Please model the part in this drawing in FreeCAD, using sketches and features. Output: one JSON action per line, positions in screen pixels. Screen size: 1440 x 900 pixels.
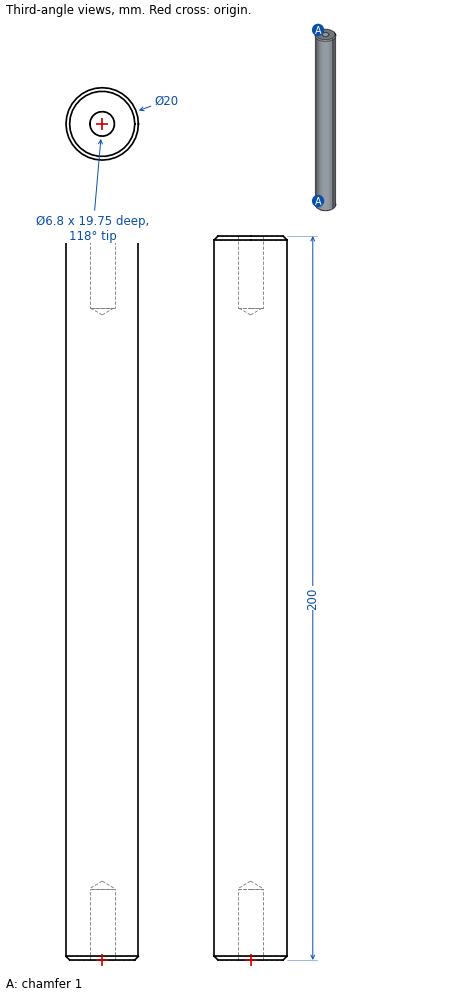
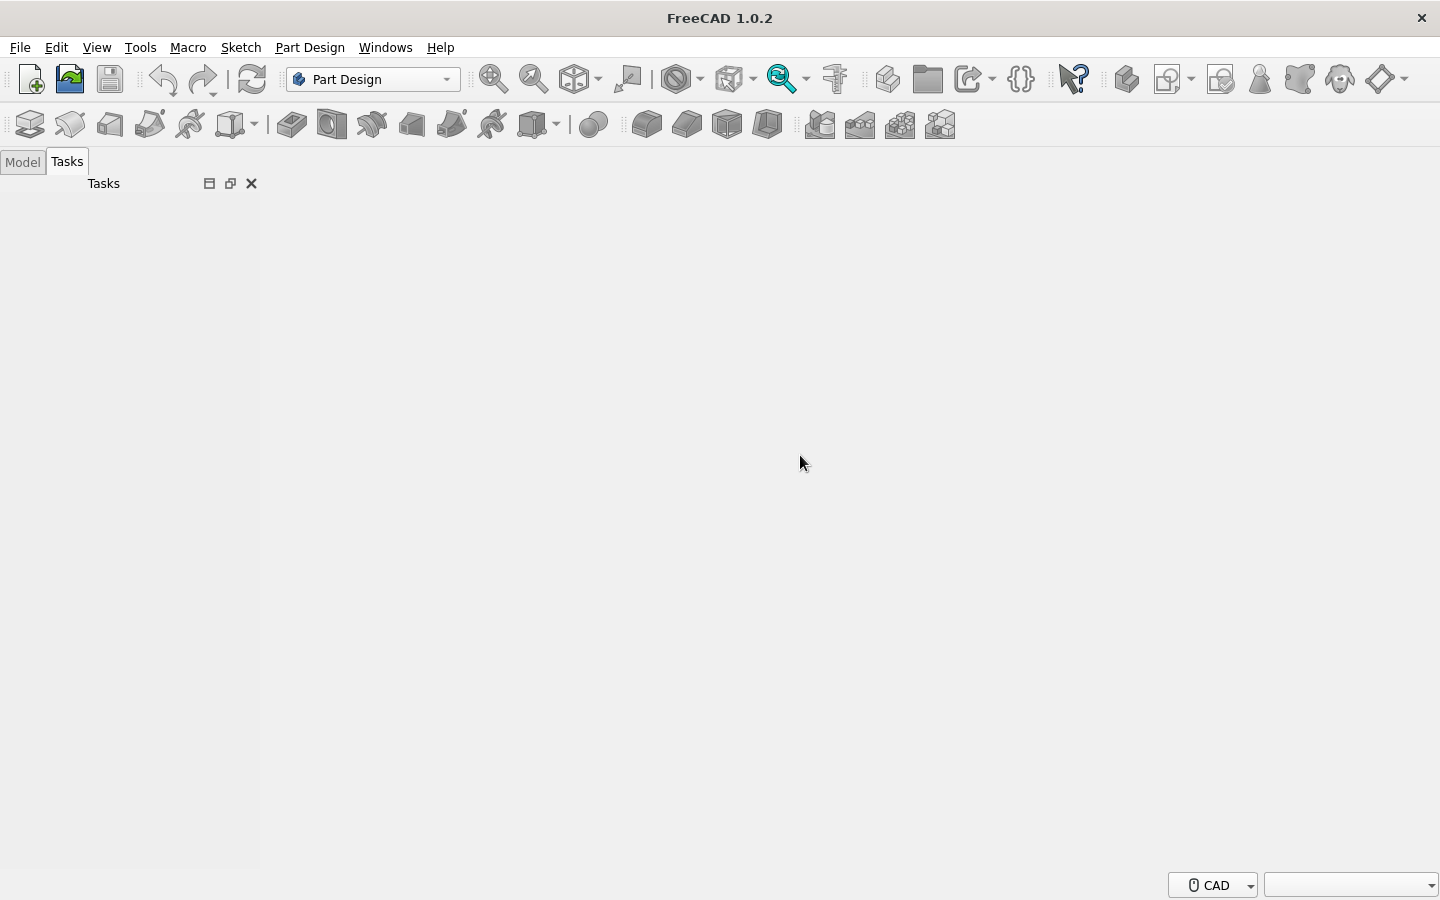
{"action": "key", "text": "ctrl+n"}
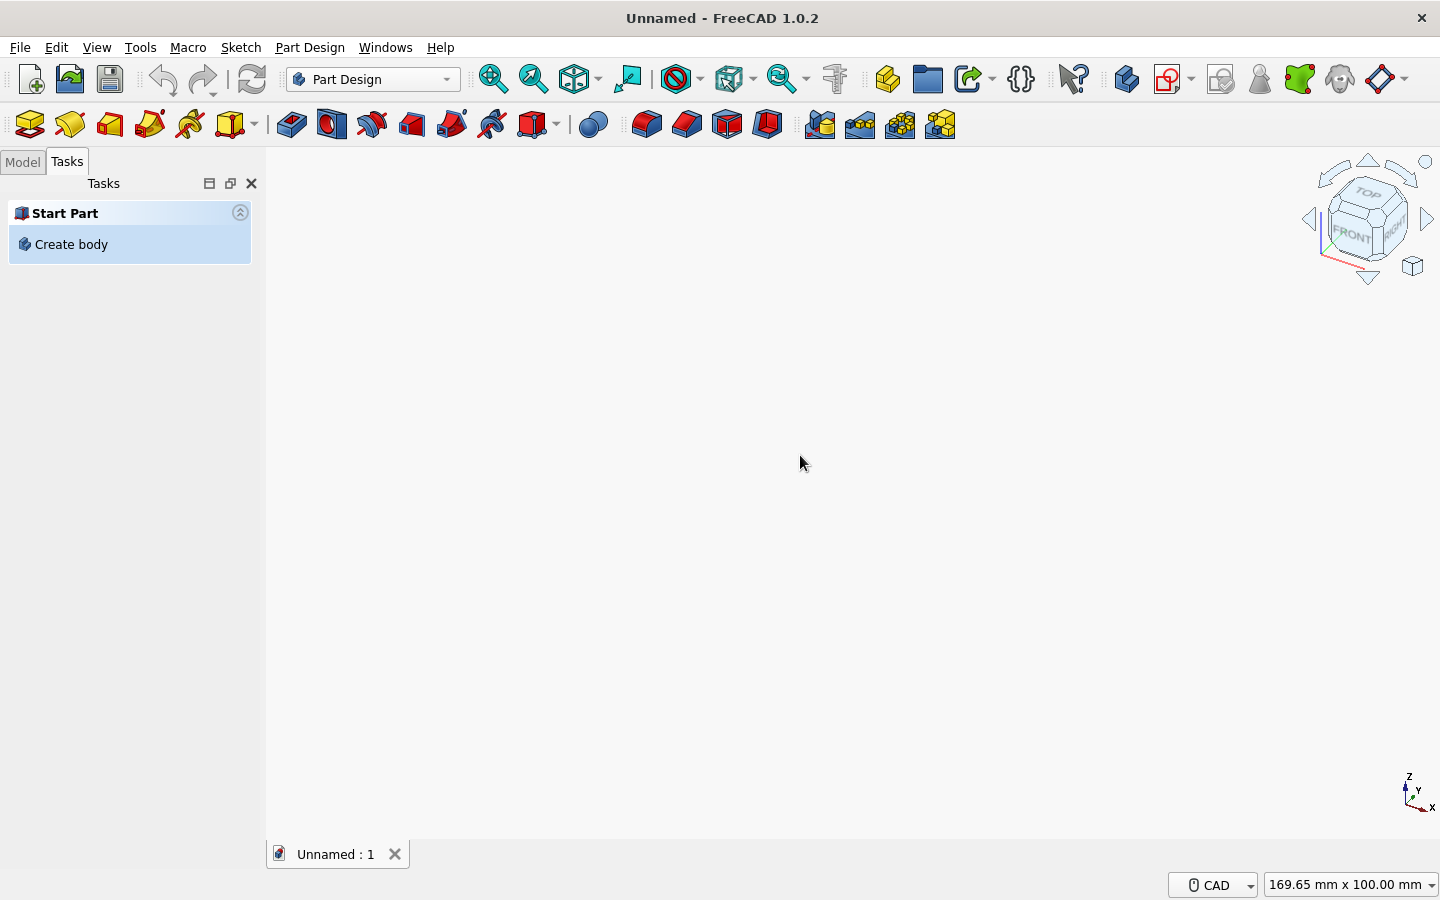
{"action": "left_click", "coordinate": [1168, 80]}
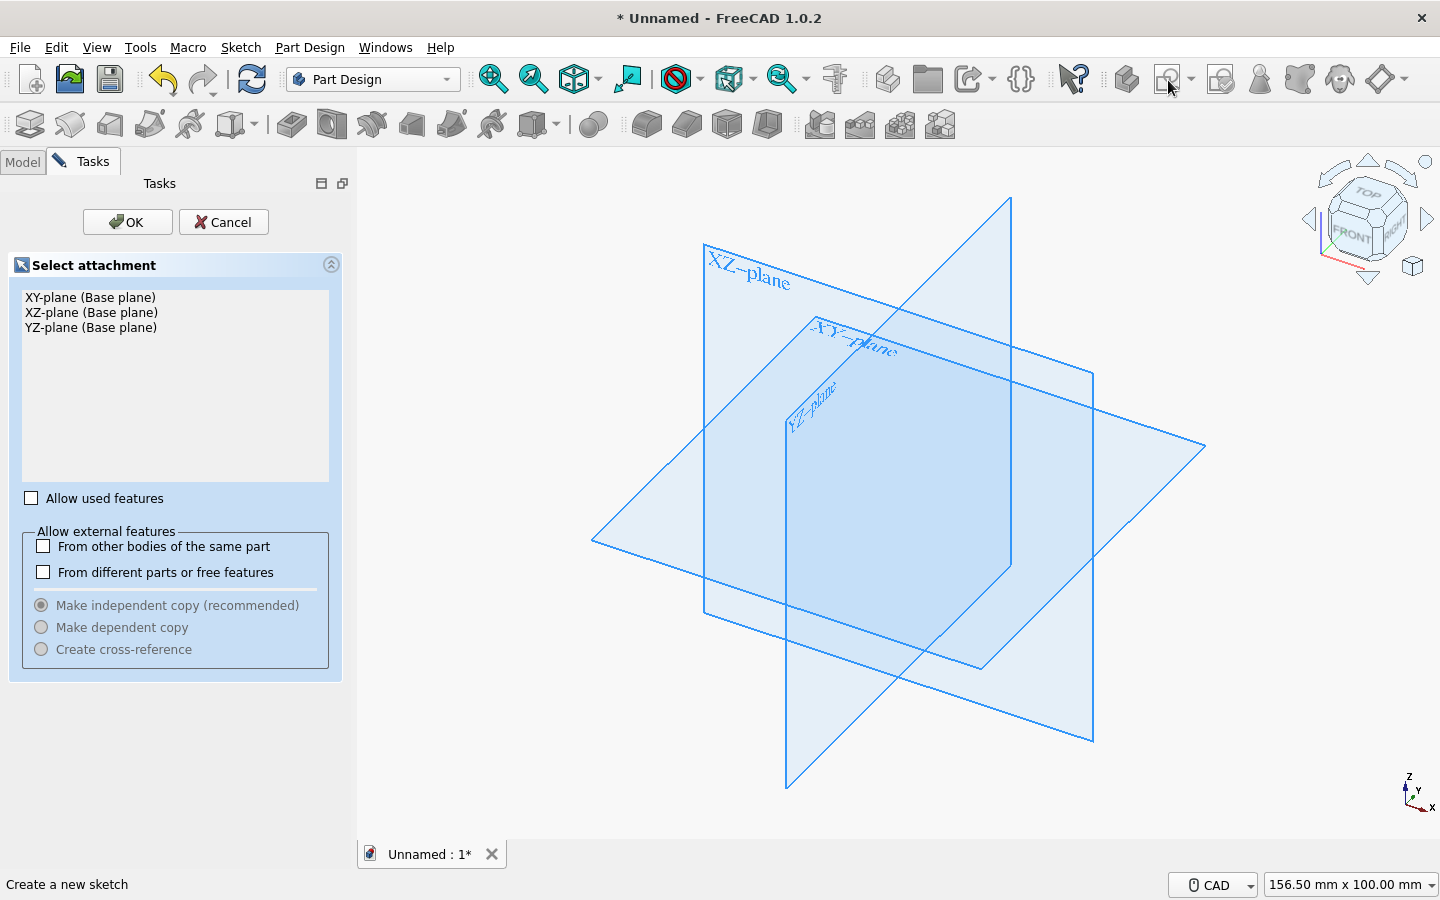
{"action": "left_click", "coordinate": [82, 298]}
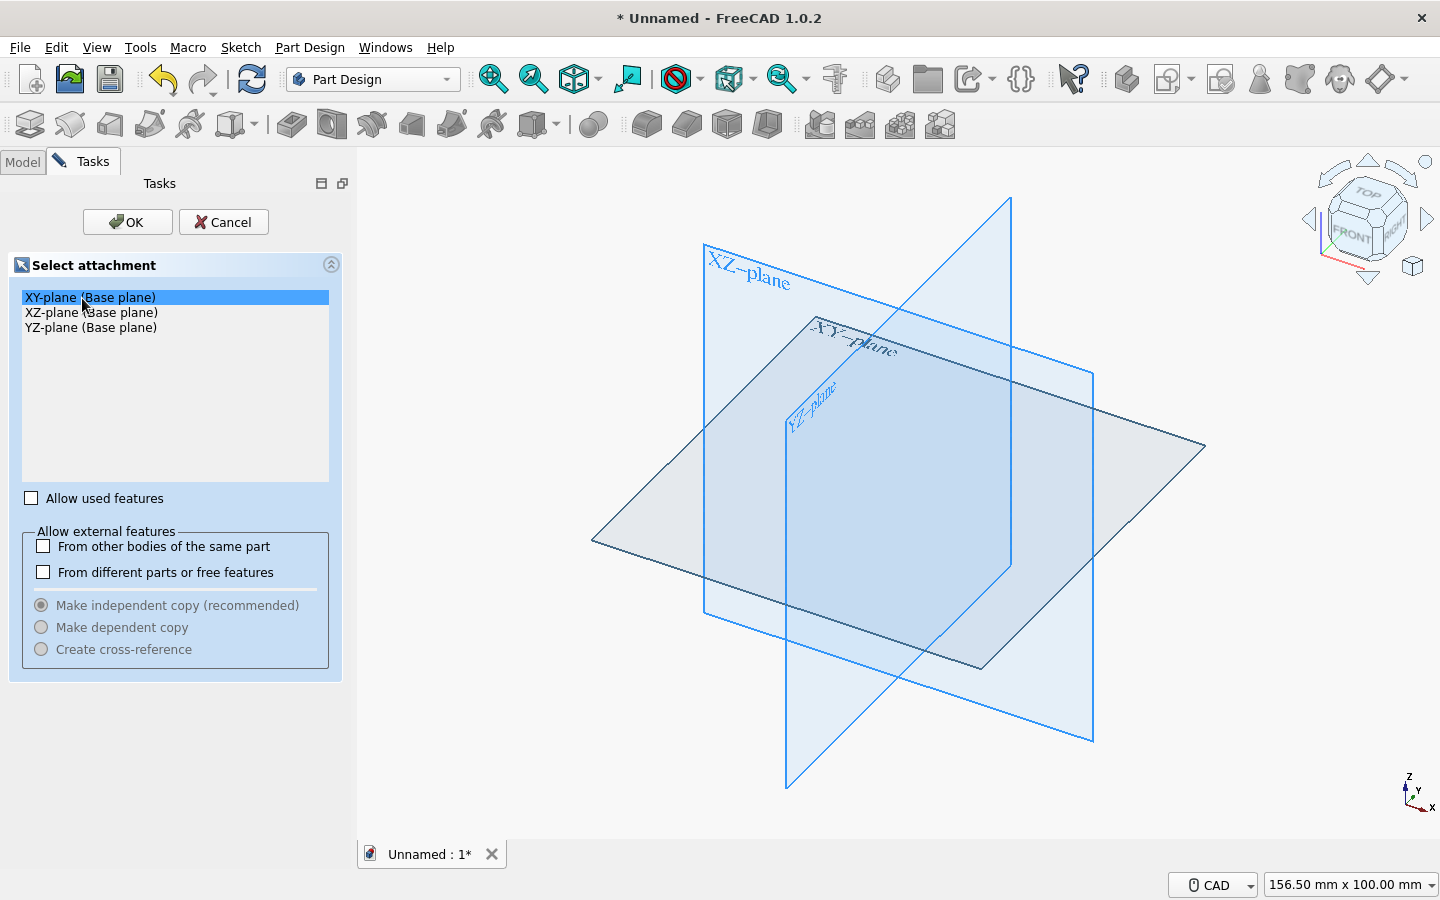
{"action": "left_click", "coordinate": [128, 222]}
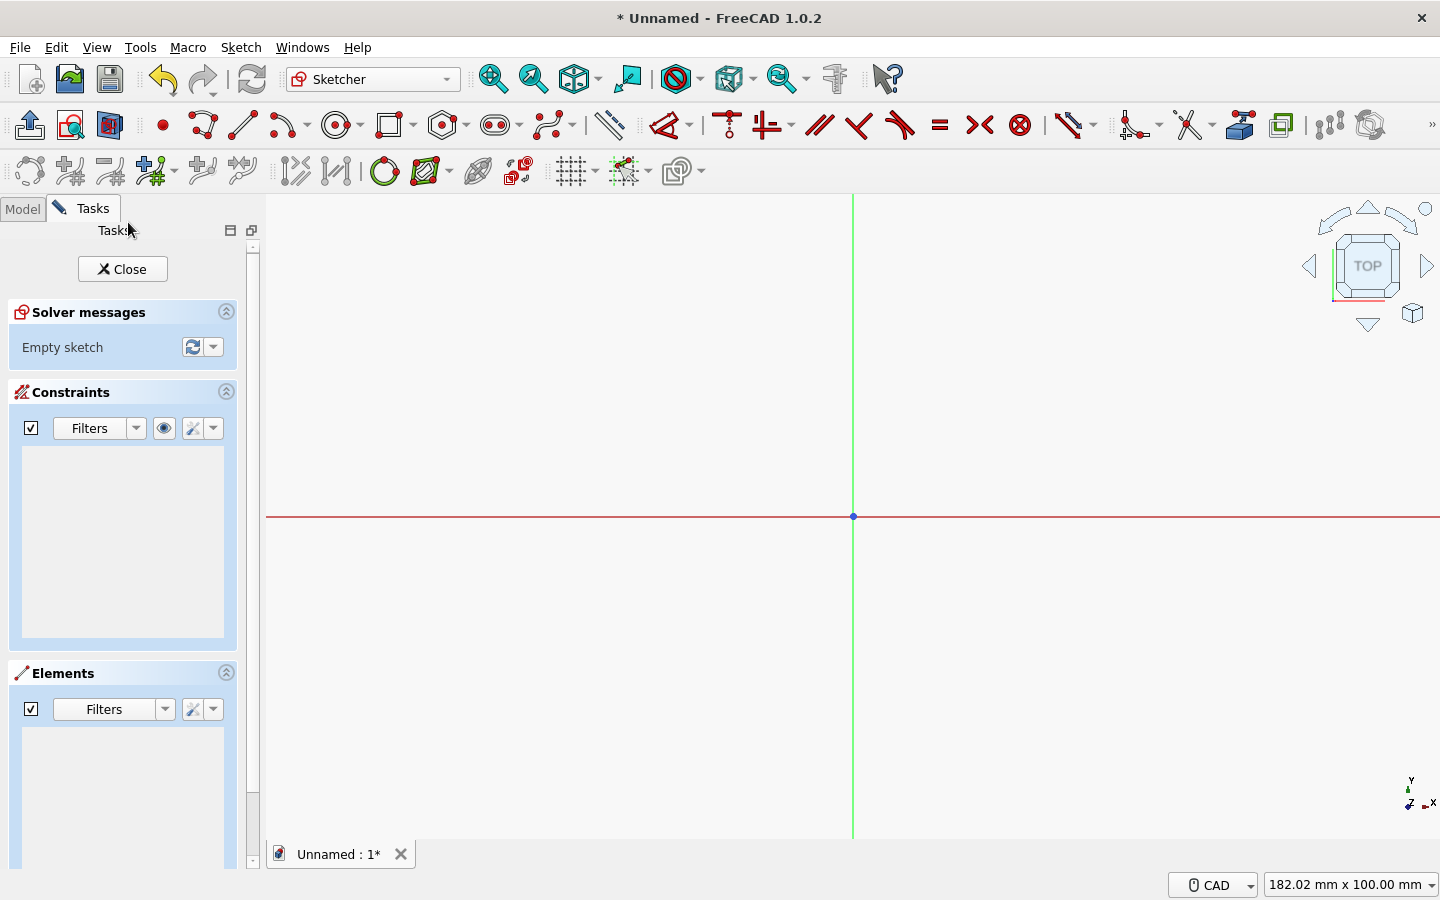
{"action": "scroll", "coordinate": [883, 516], "scroll_direction": "up", "scroll_amount": 6}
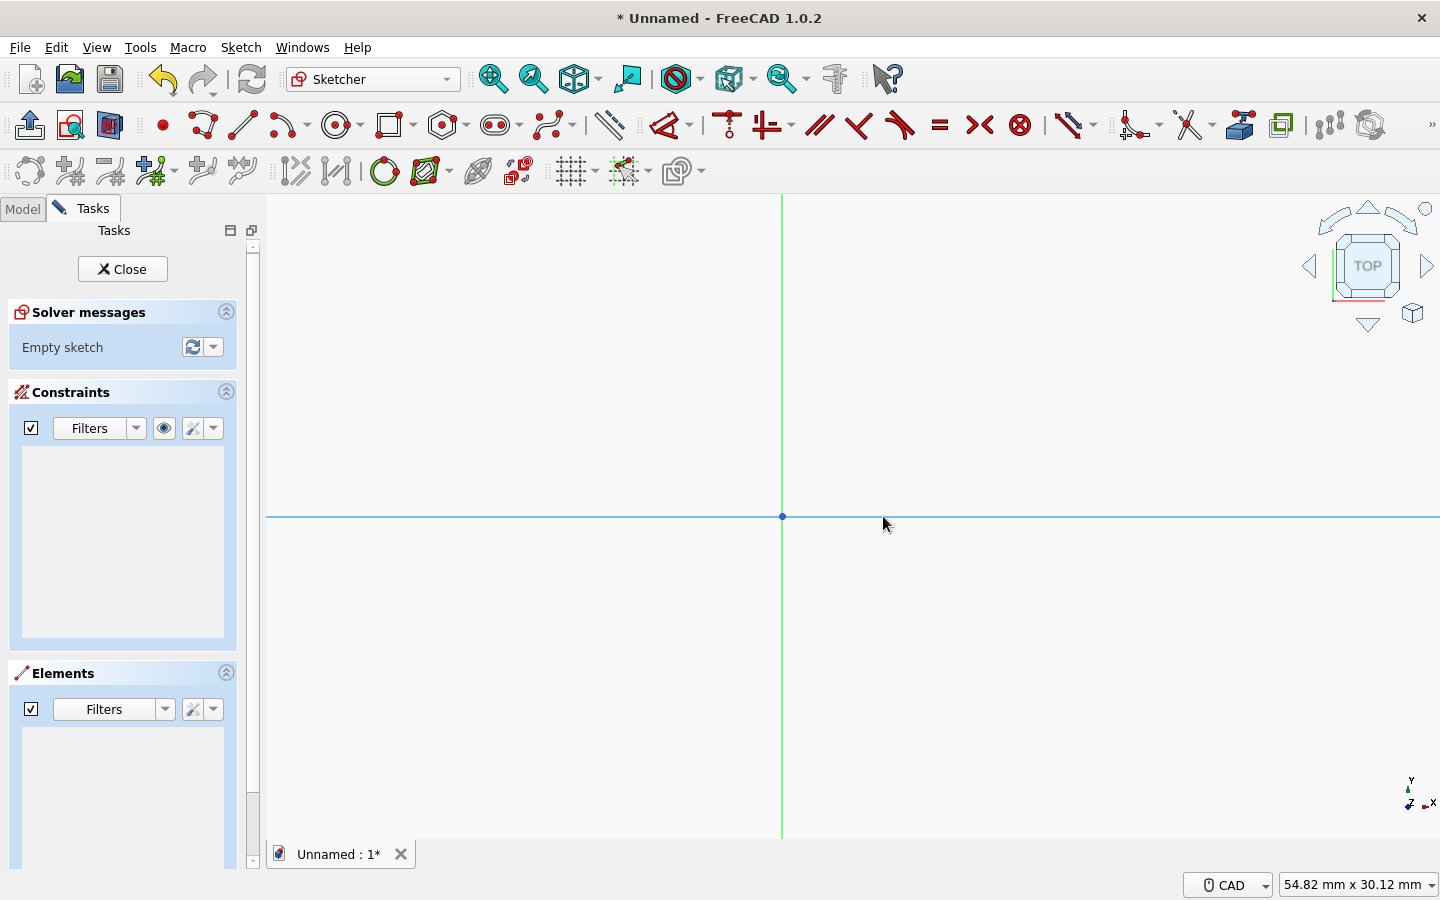
{"action": "key", "text": "g c"}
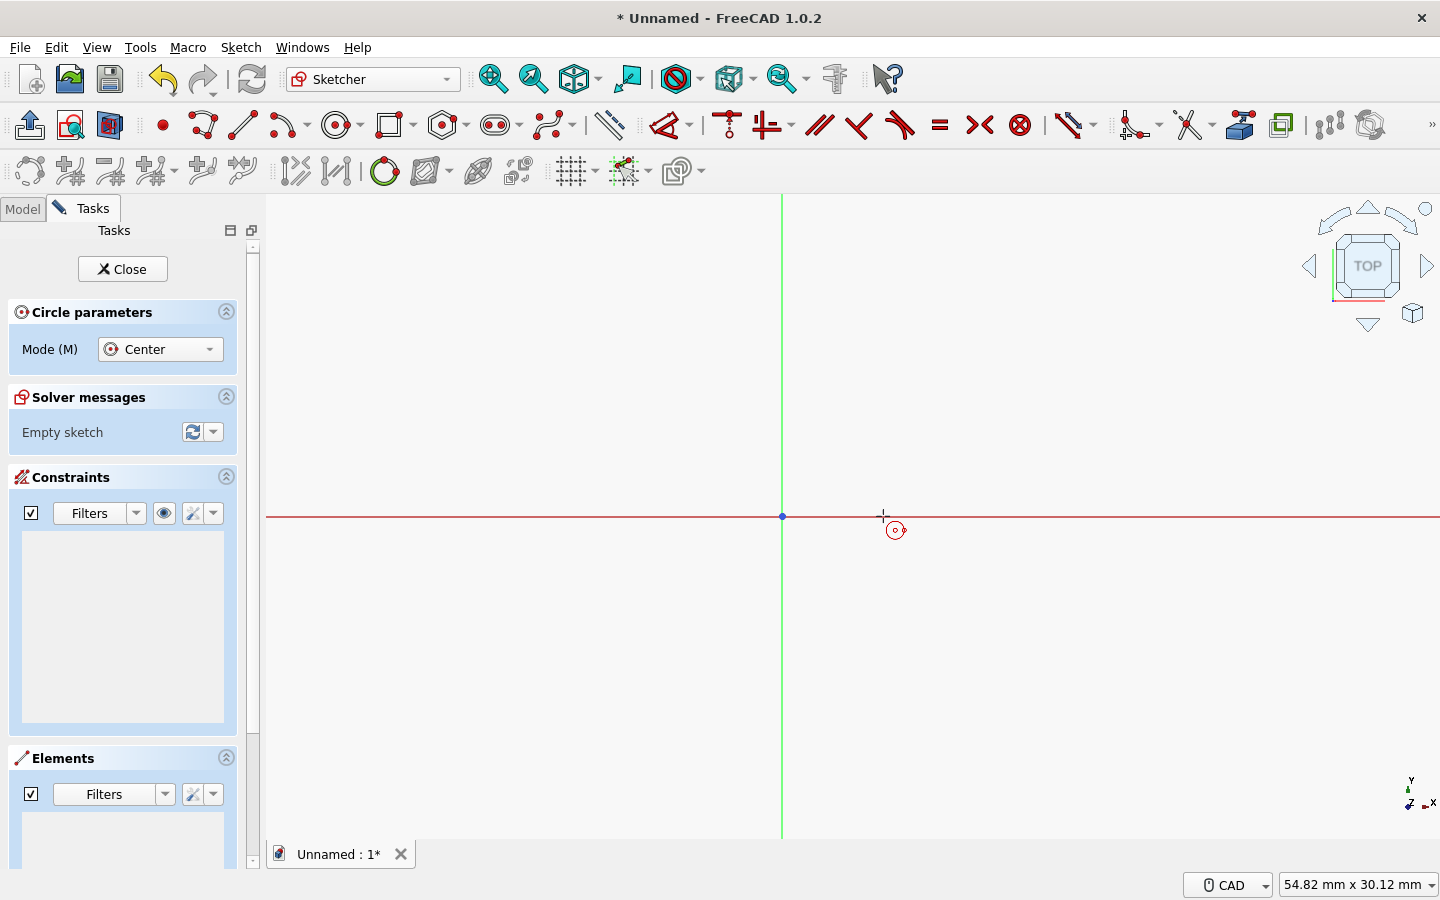
{"action": "left_click", "coordinate": [782, 516]}
{"action": "mouse_move", "coordinate": [934, 365]}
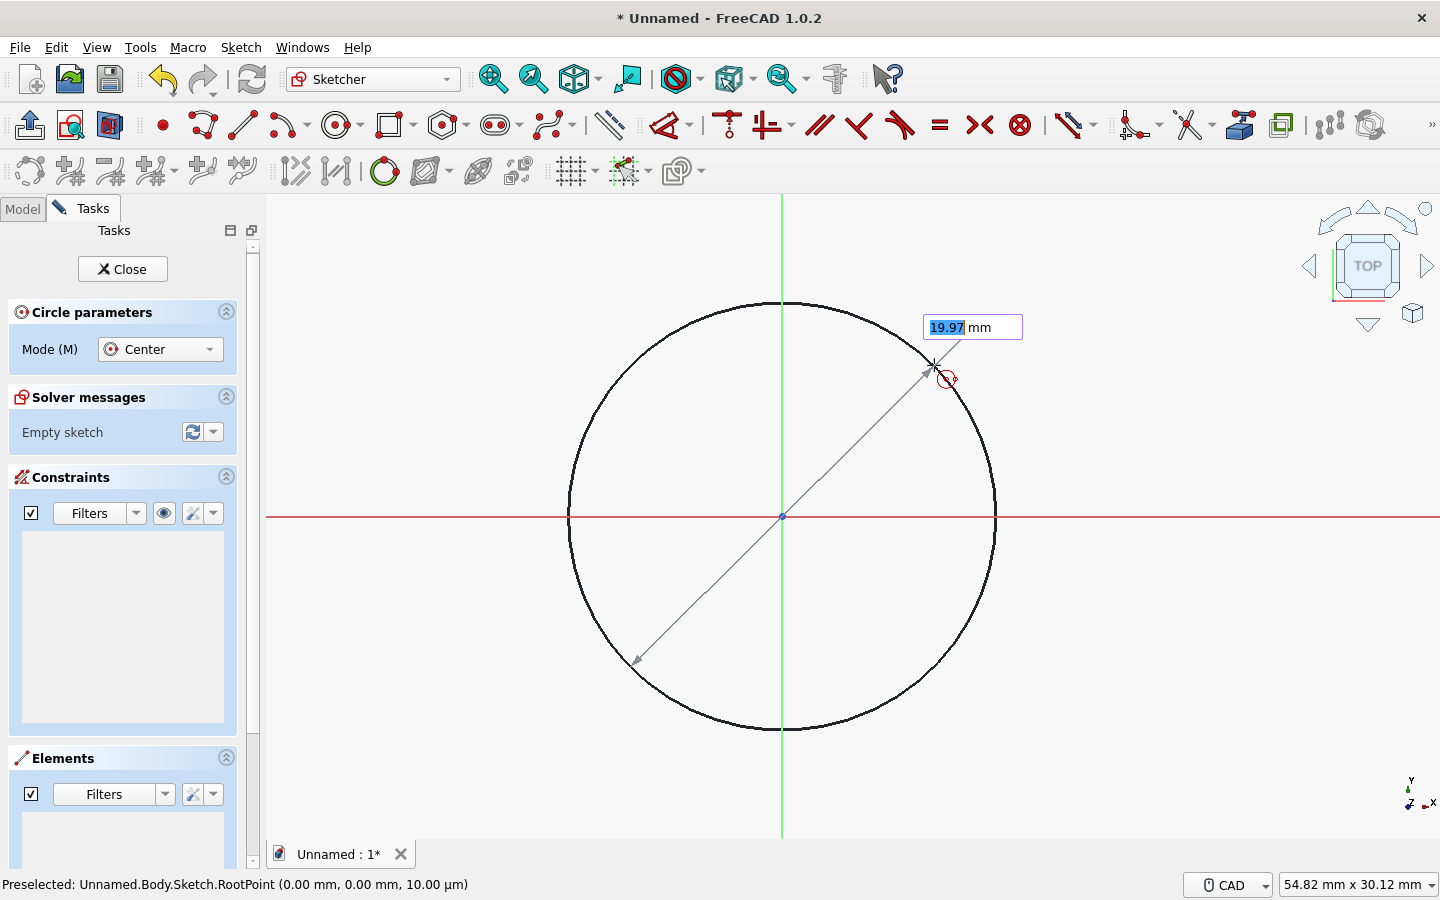
{"action": "type", "text": "20"}
{"action": "key", "text": "Return"}
{"action": "key", "text": "Escape"}